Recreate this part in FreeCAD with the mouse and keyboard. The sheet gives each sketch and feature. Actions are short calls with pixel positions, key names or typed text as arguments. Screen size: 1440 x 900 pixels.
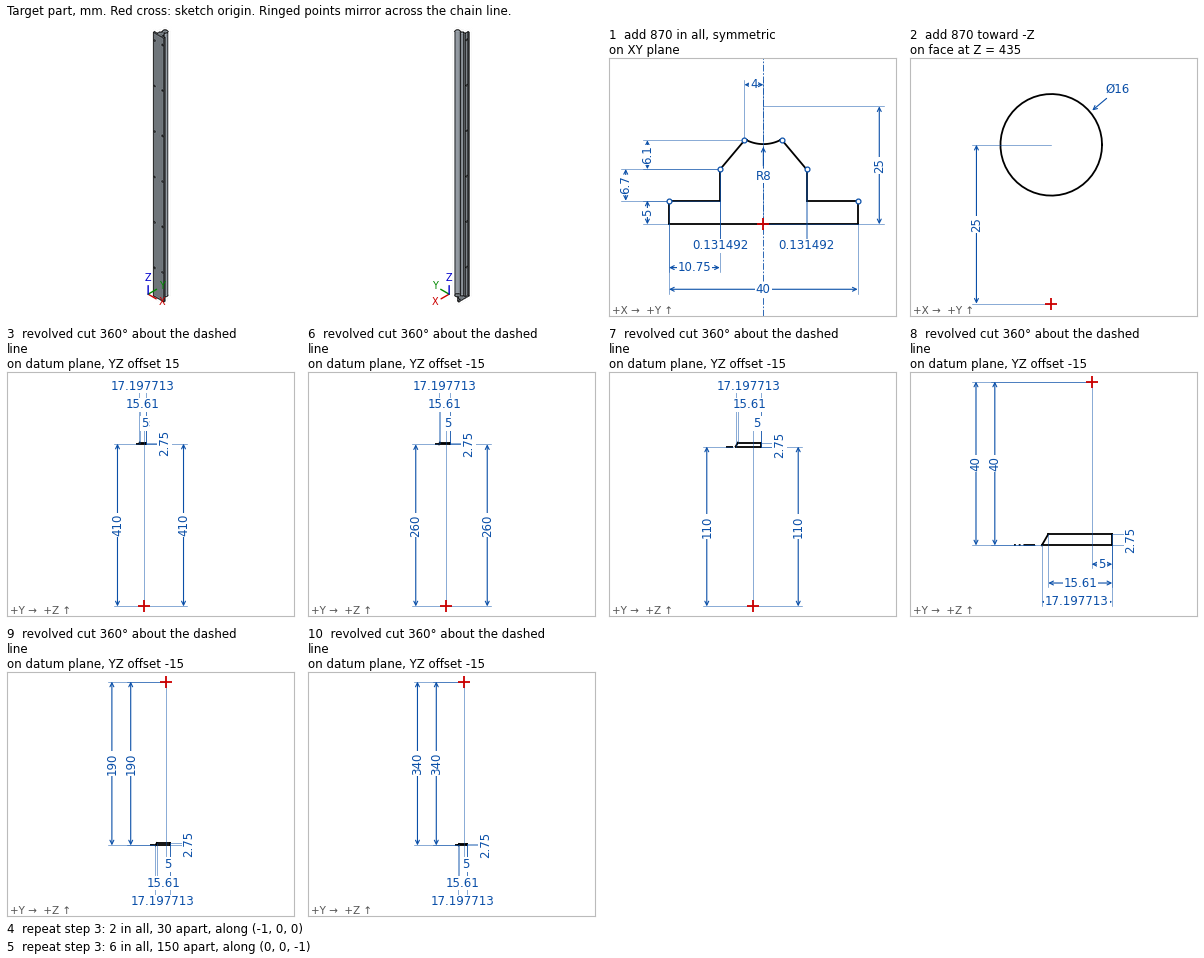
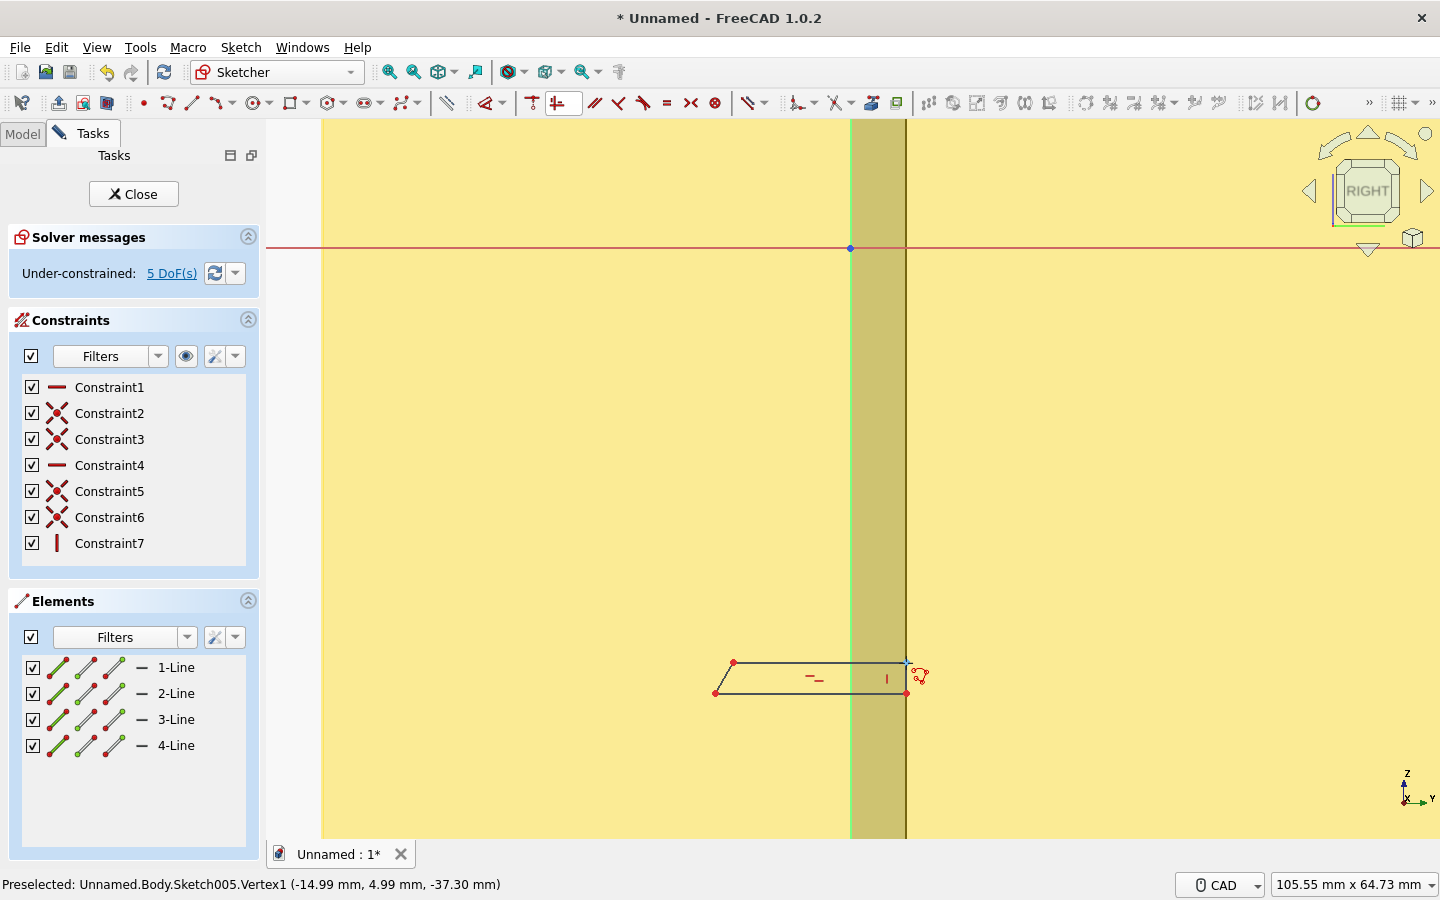
key(g)
key(l)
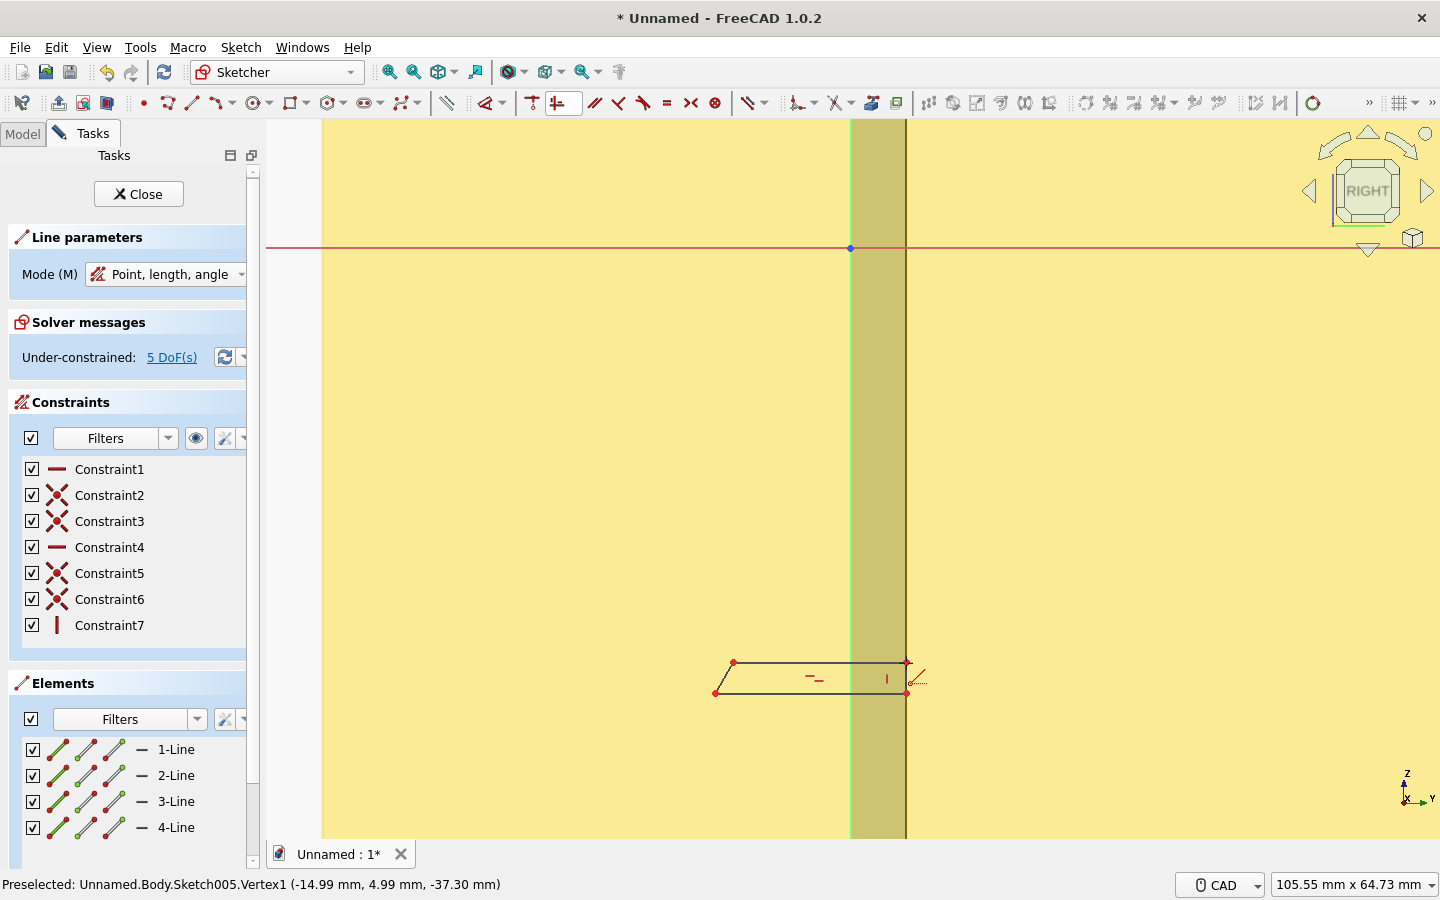
click(696, 693)
click(638, 693)
key(Escape)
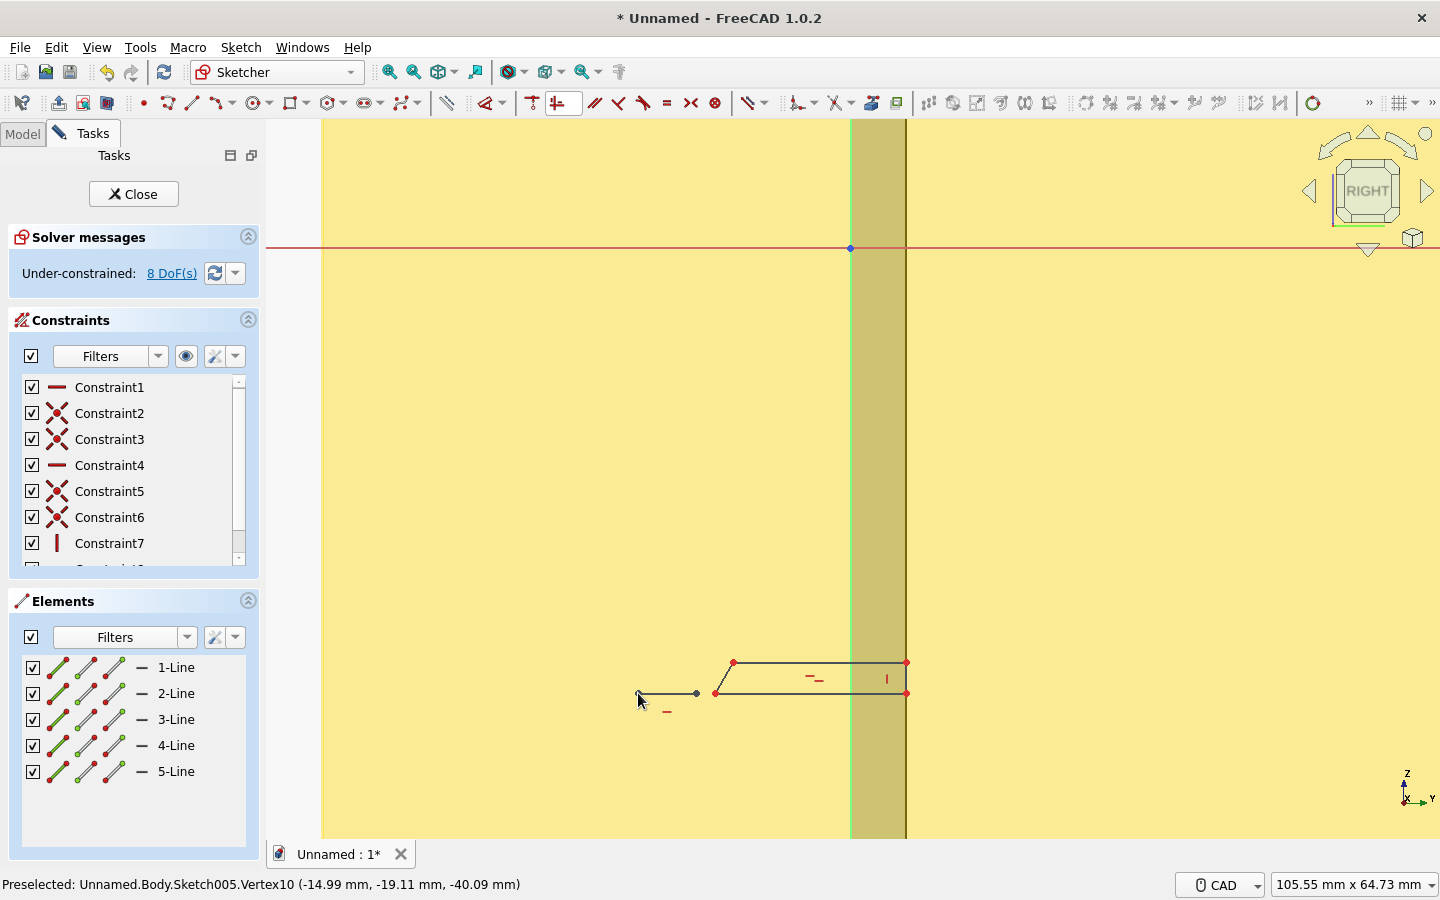
click(679, 694)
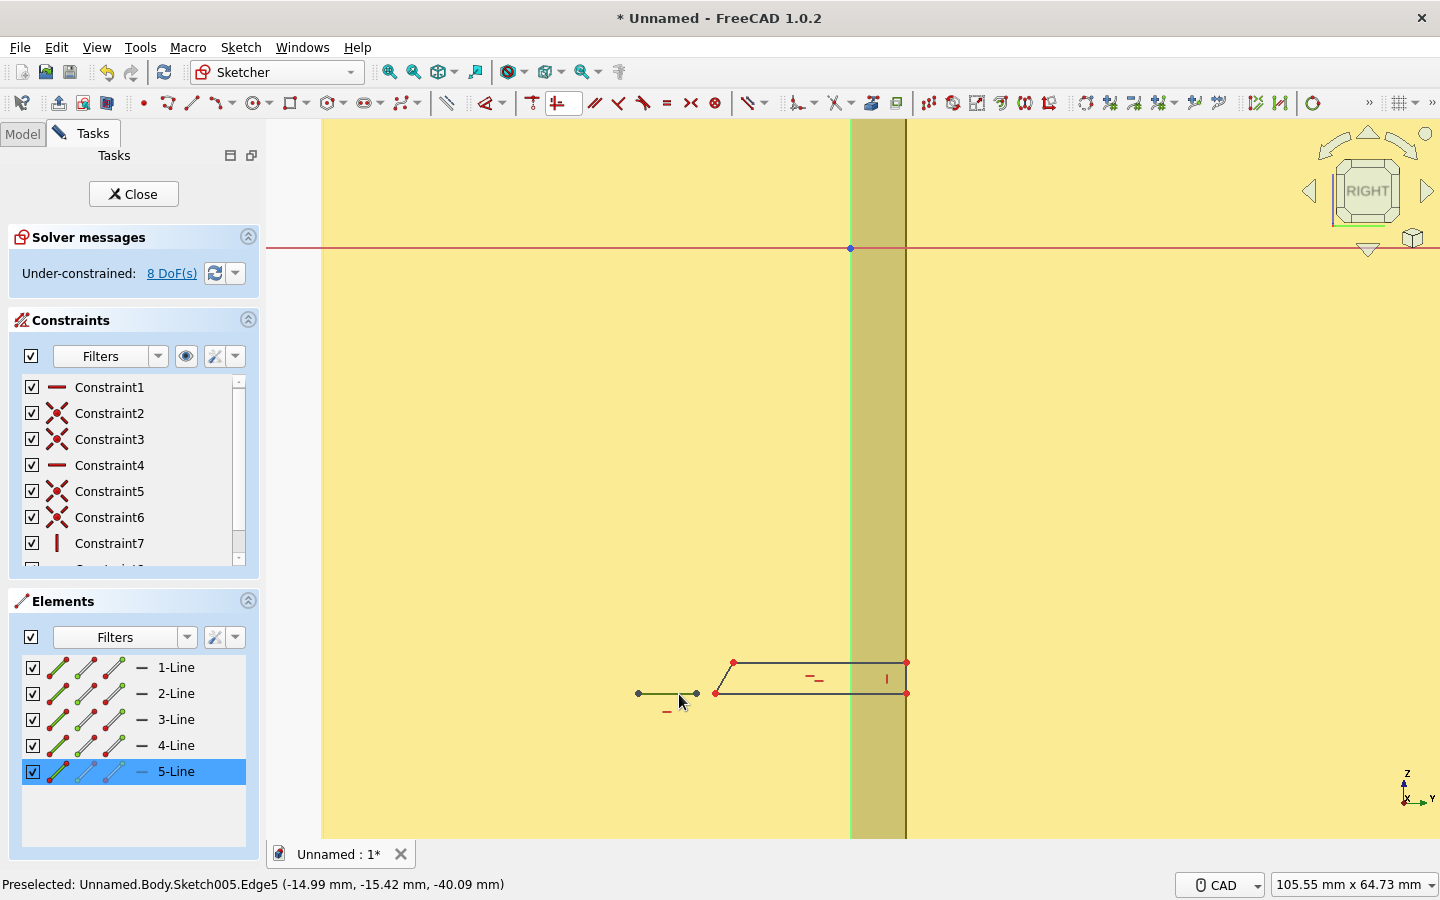
click(448, 104)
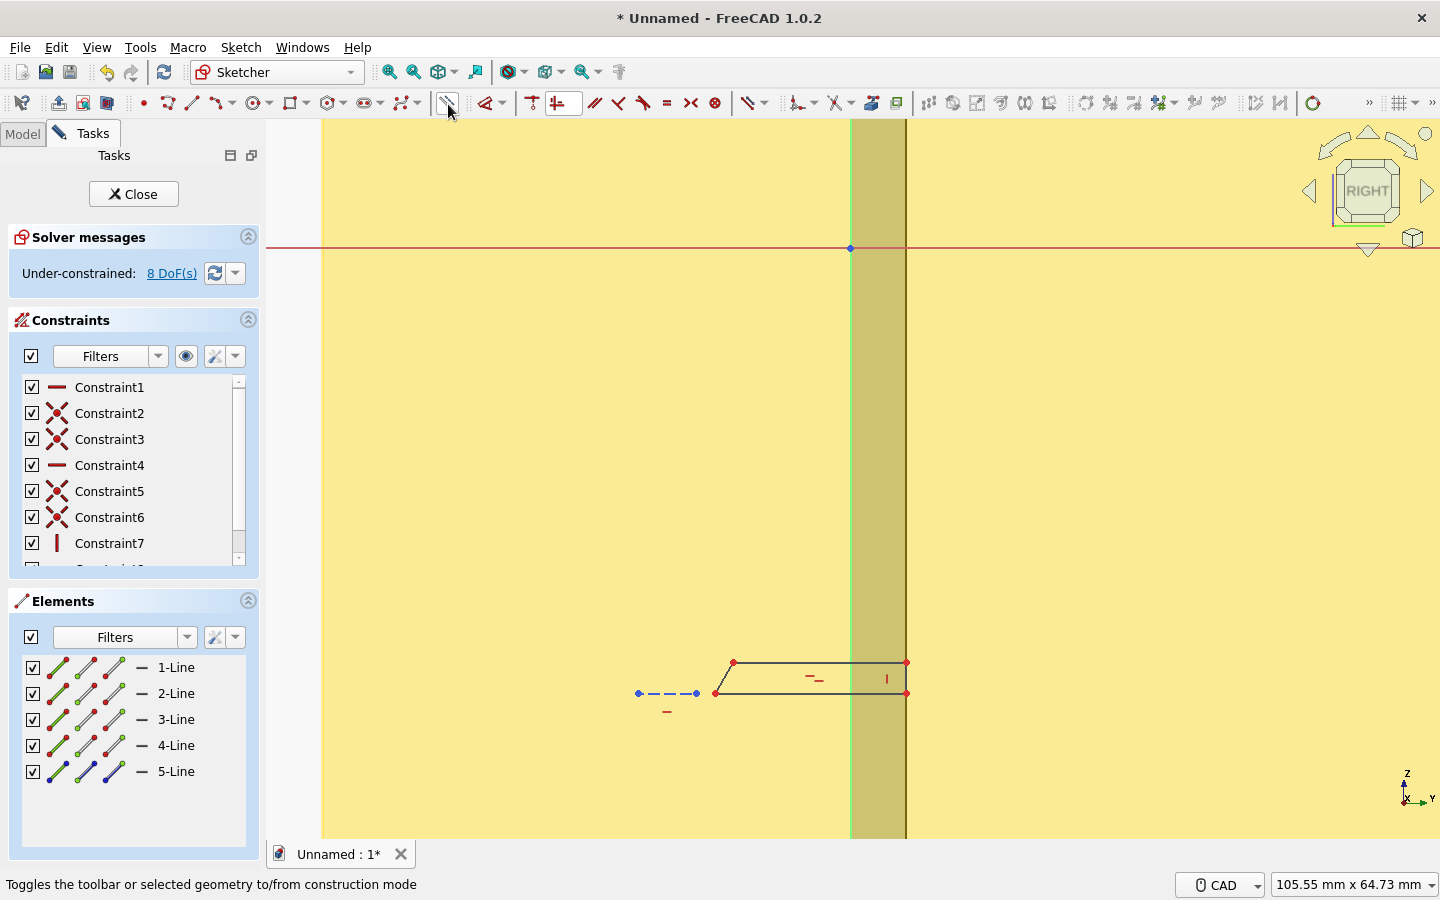
click(486, 104)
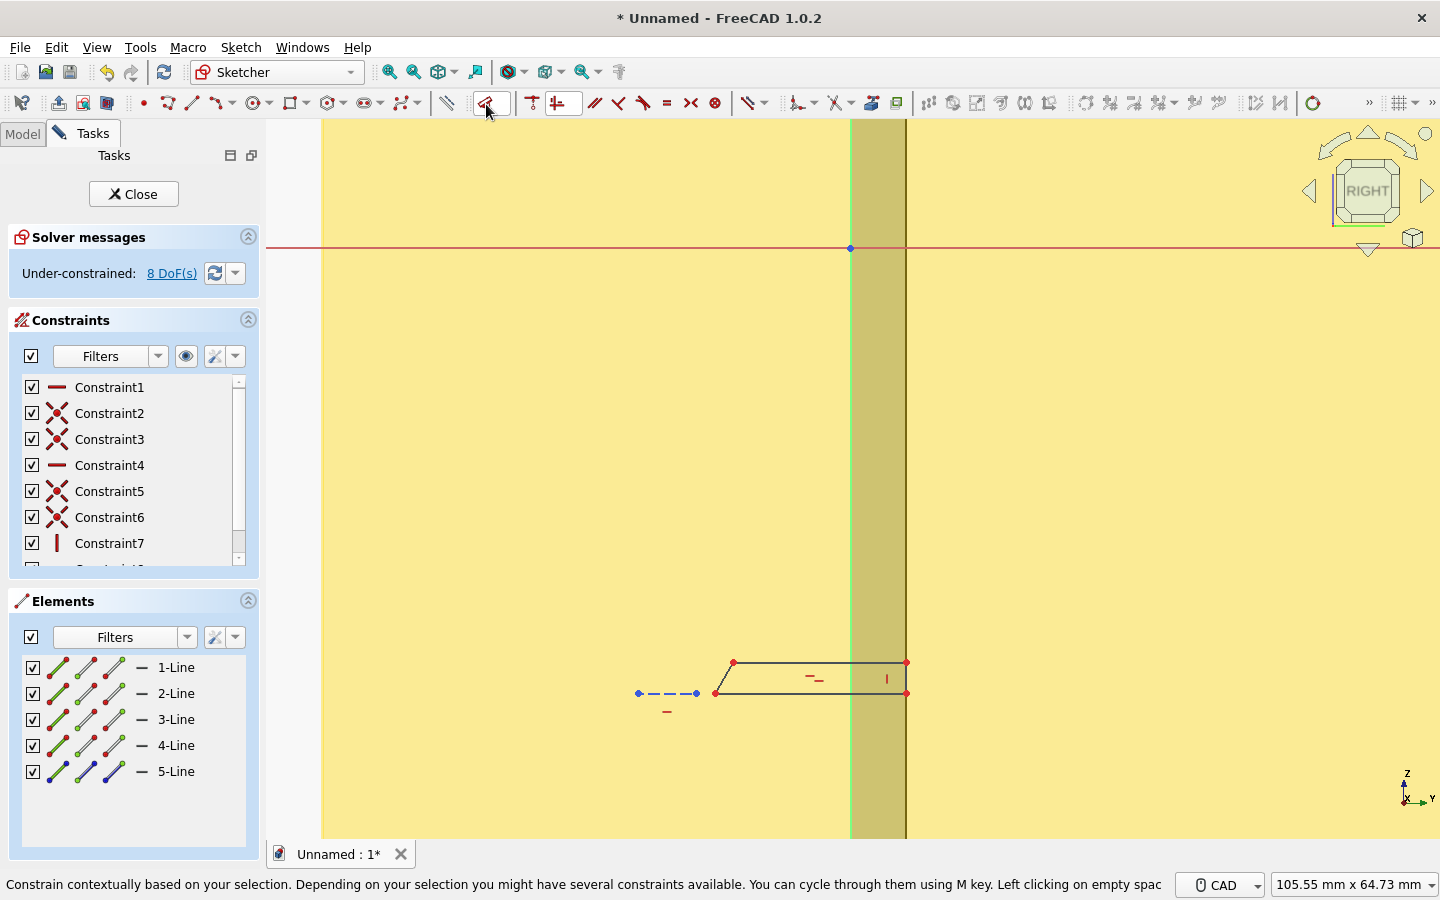
click(906, 663)
click(878, 214)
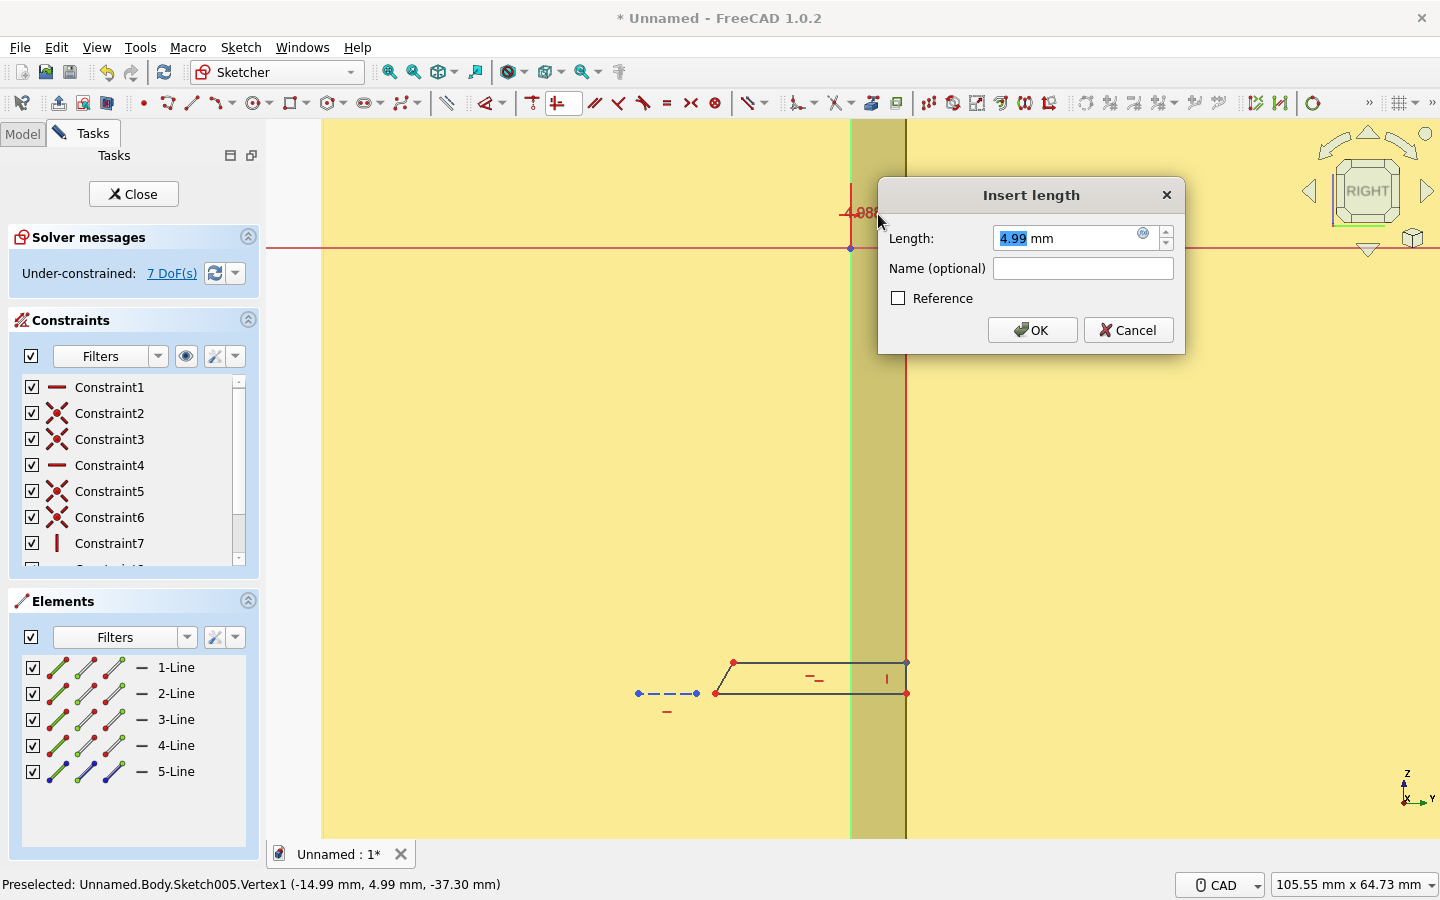
text(5)
key(Return)